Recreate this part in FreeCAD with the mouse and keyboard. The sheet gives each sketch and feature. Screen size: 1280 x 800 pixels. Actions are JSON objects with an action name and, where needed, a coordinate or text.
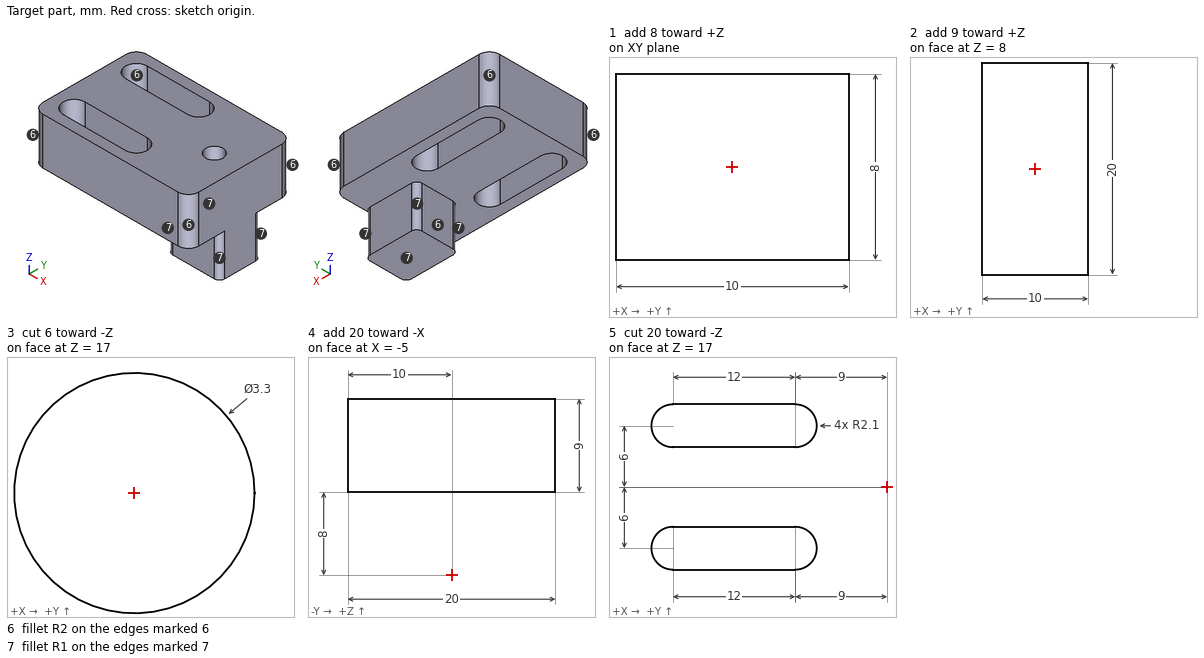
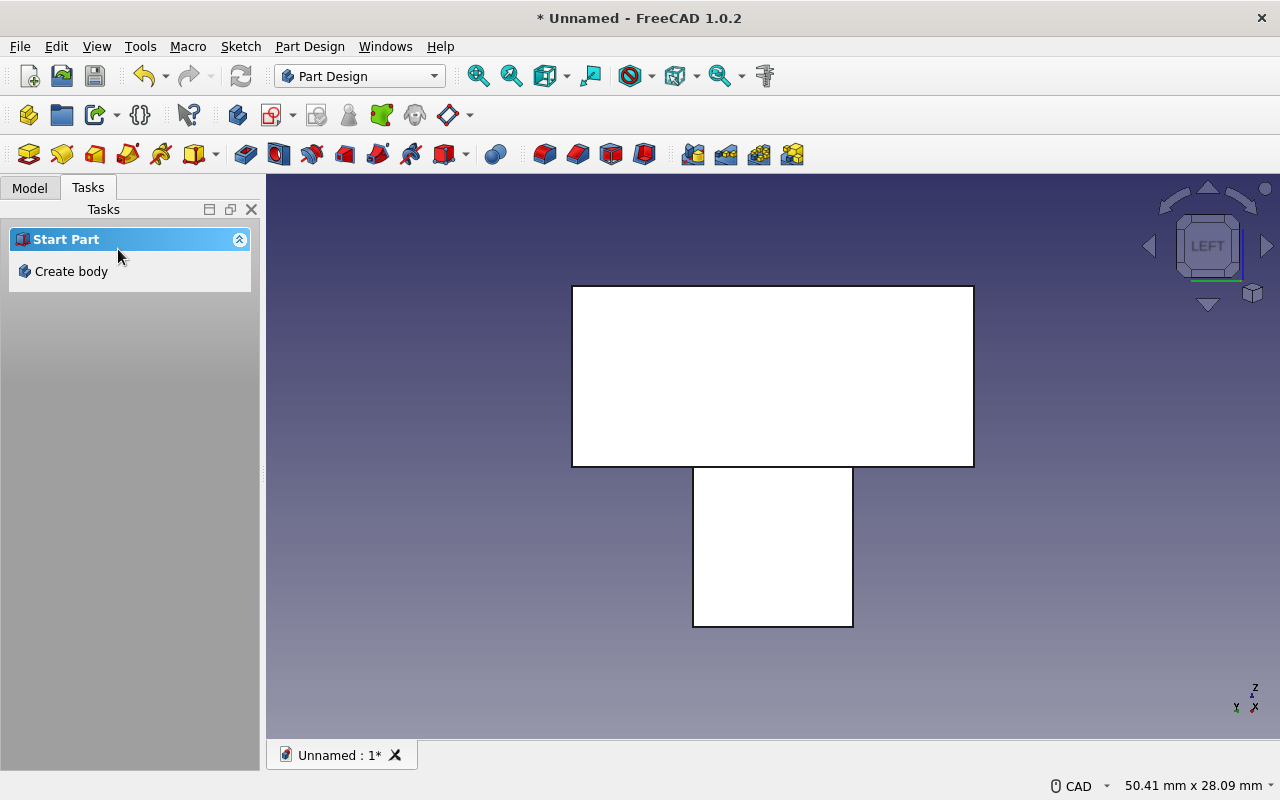
{"action": "key", "text": "0"}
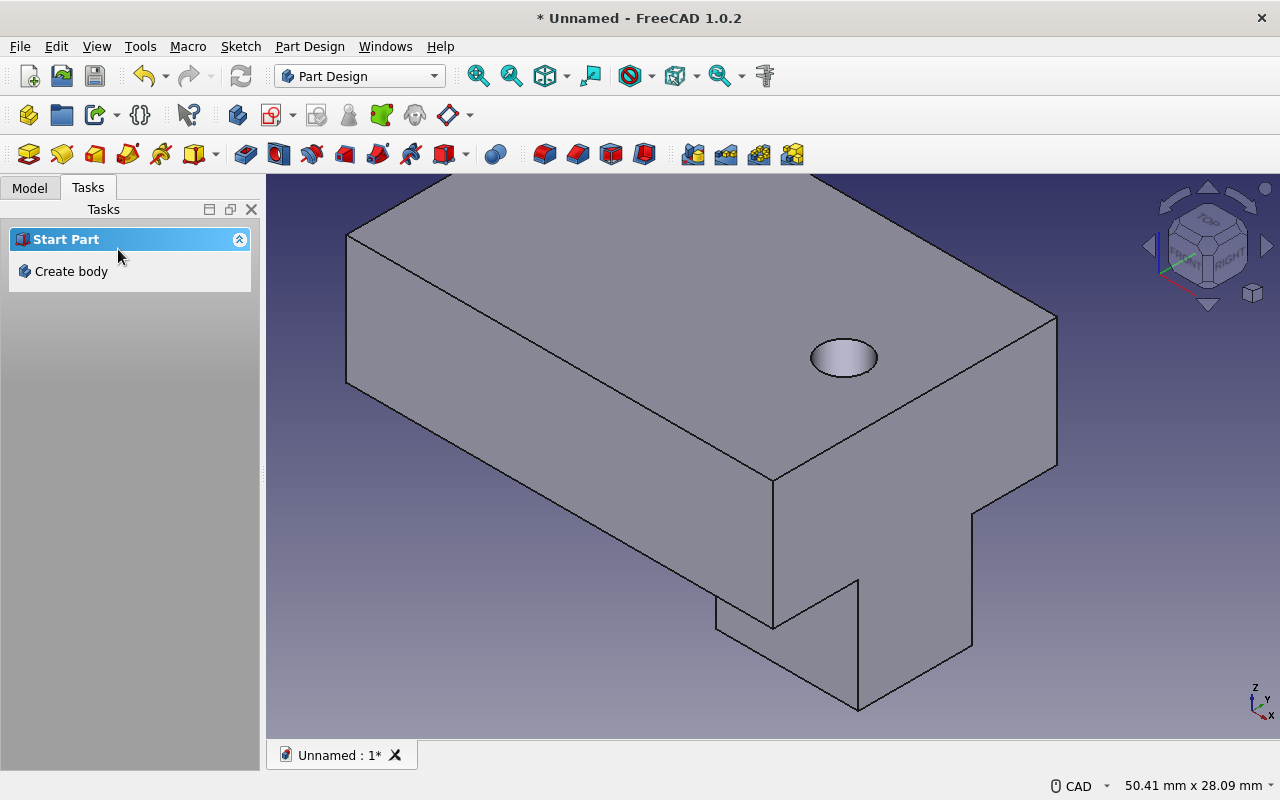
{"action": "left_click", "coordinate": [479, 76]}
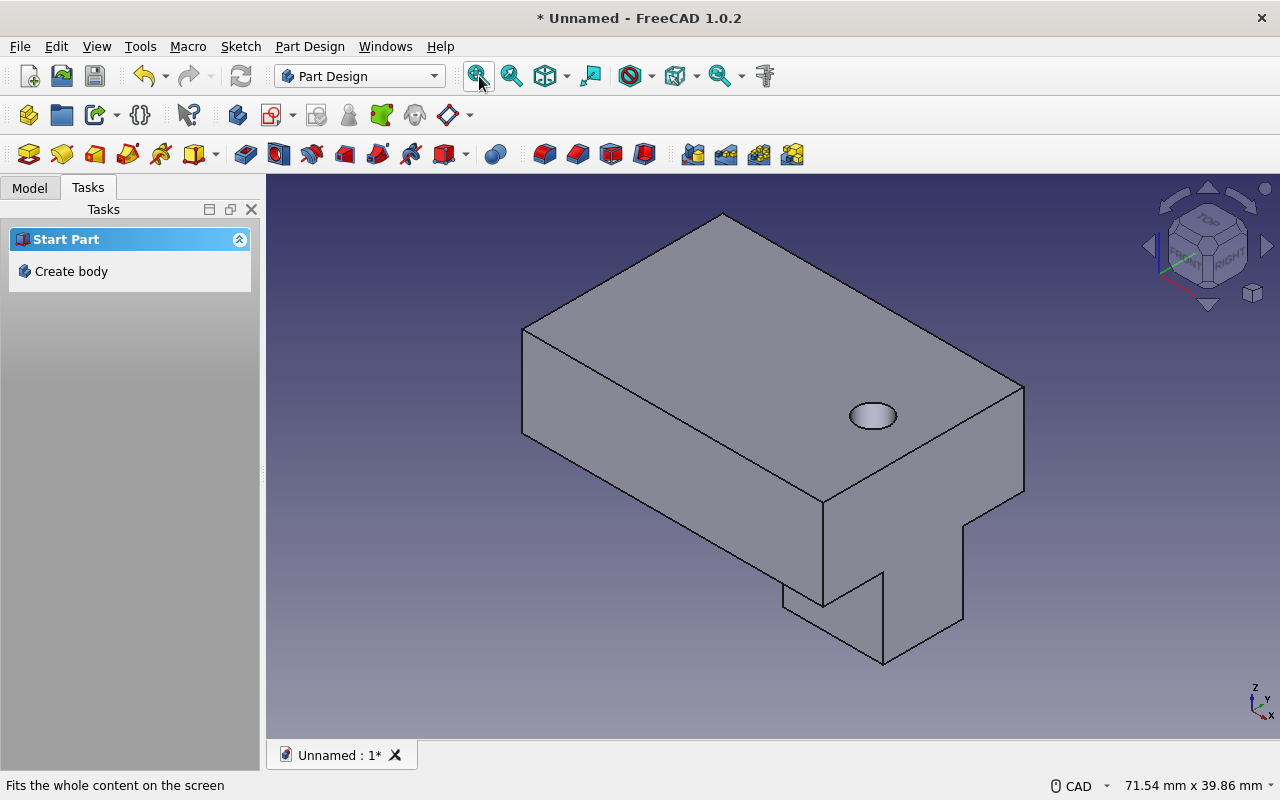
{"action": "left_click", "coordinate": [730, 332]}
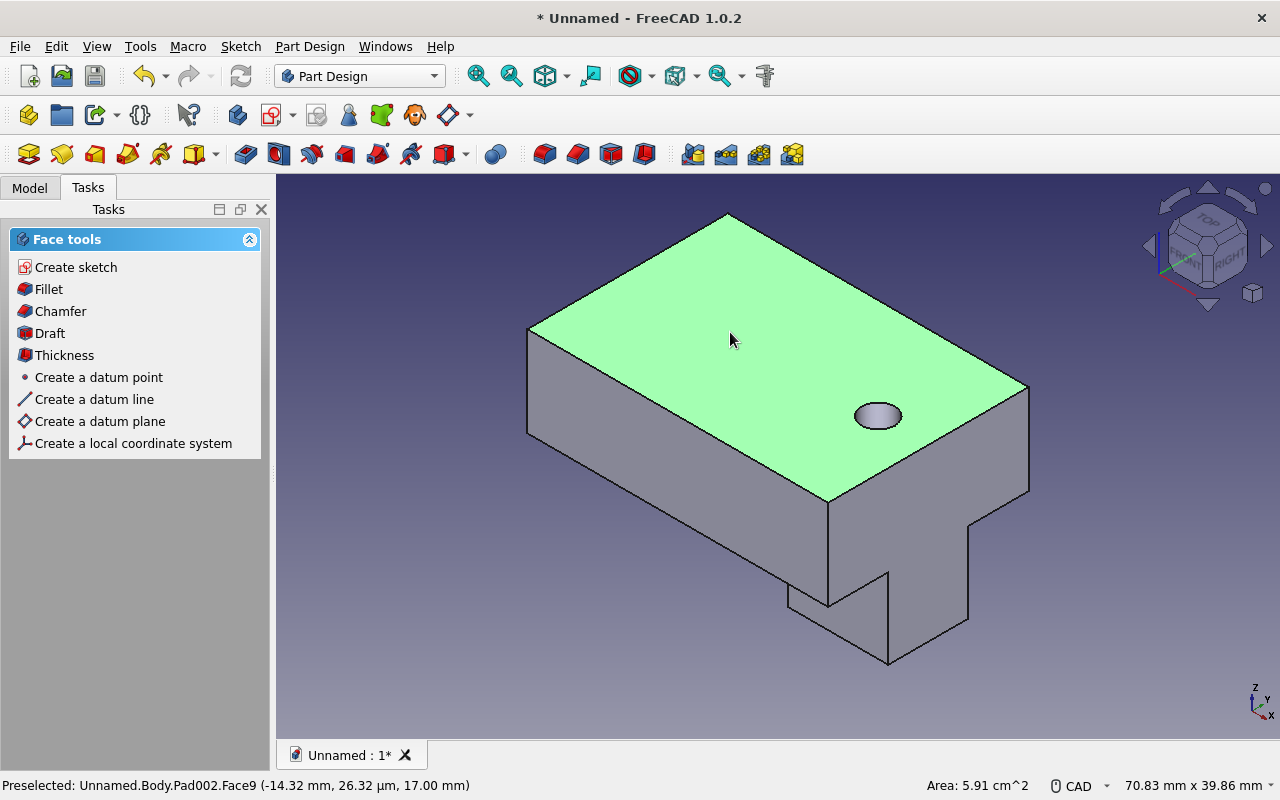
{"action": "left_click", "coordinate": [270, 116]}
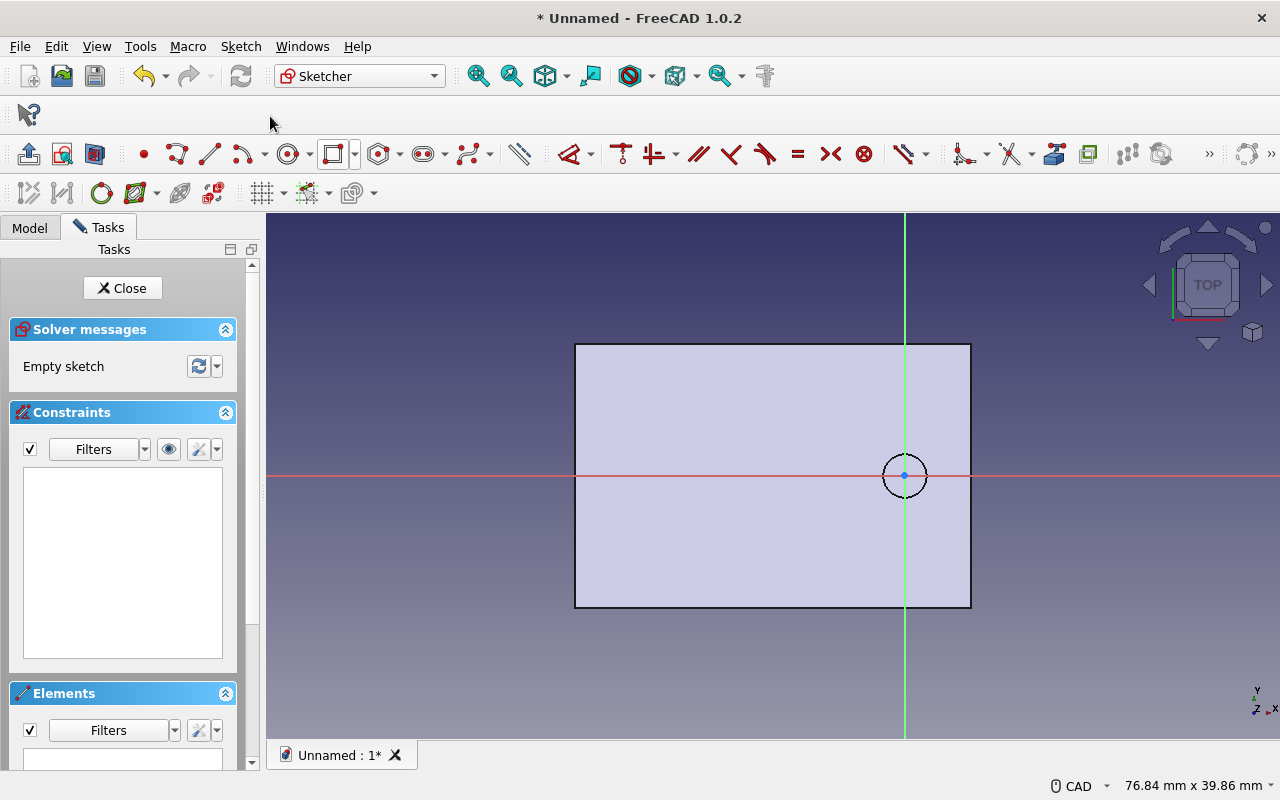
{"action": "scroll", "coordinate": [850, 476], "scroll_direction": "up", "scroll_amount": 2}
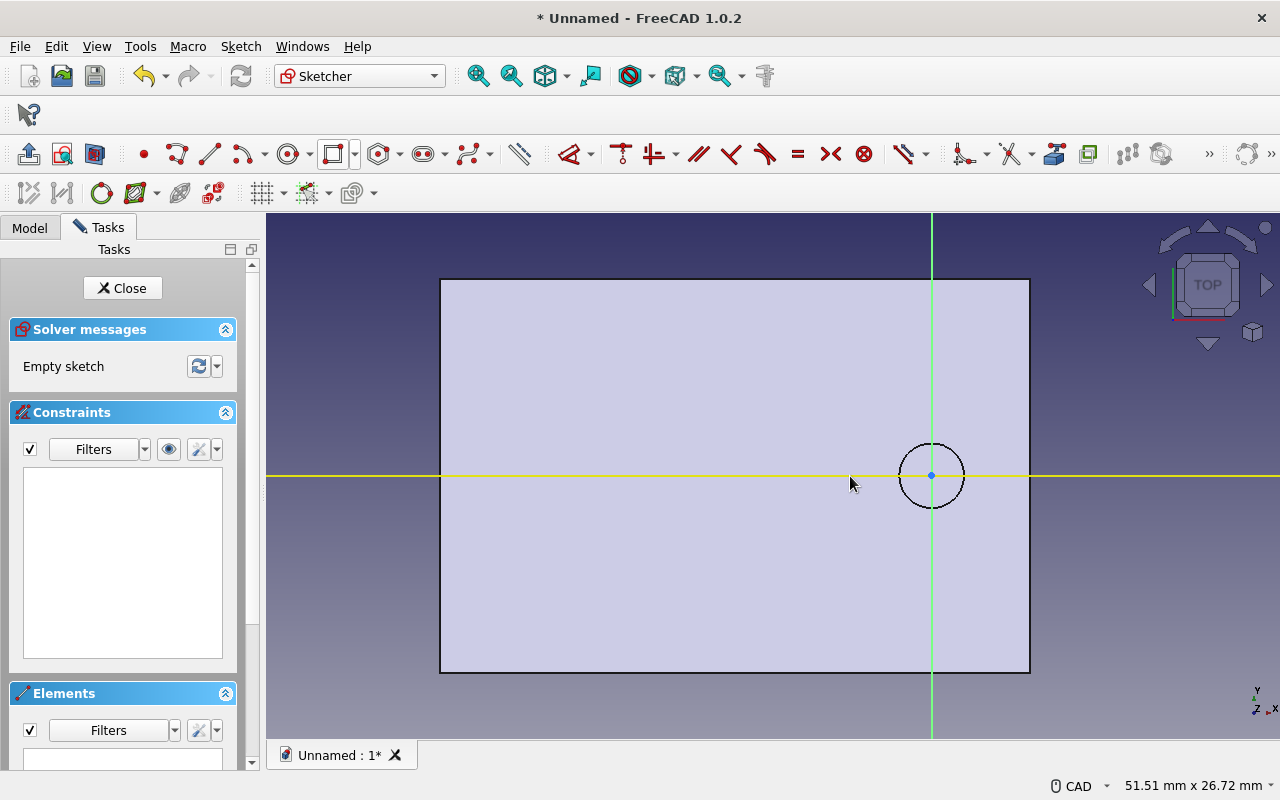
{"action": "left_click", "coordinate": [422, 154]}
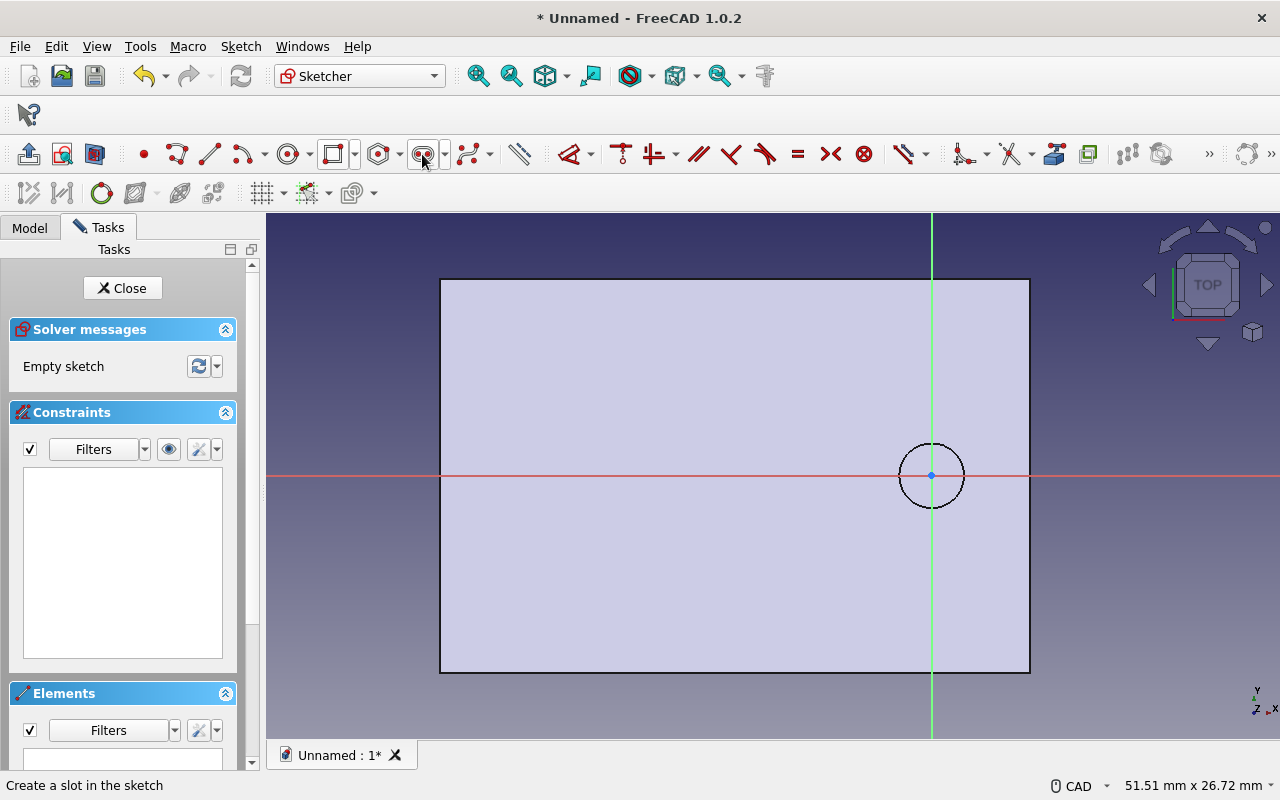
{"action": "left_click", "coordinate": [518, 358]}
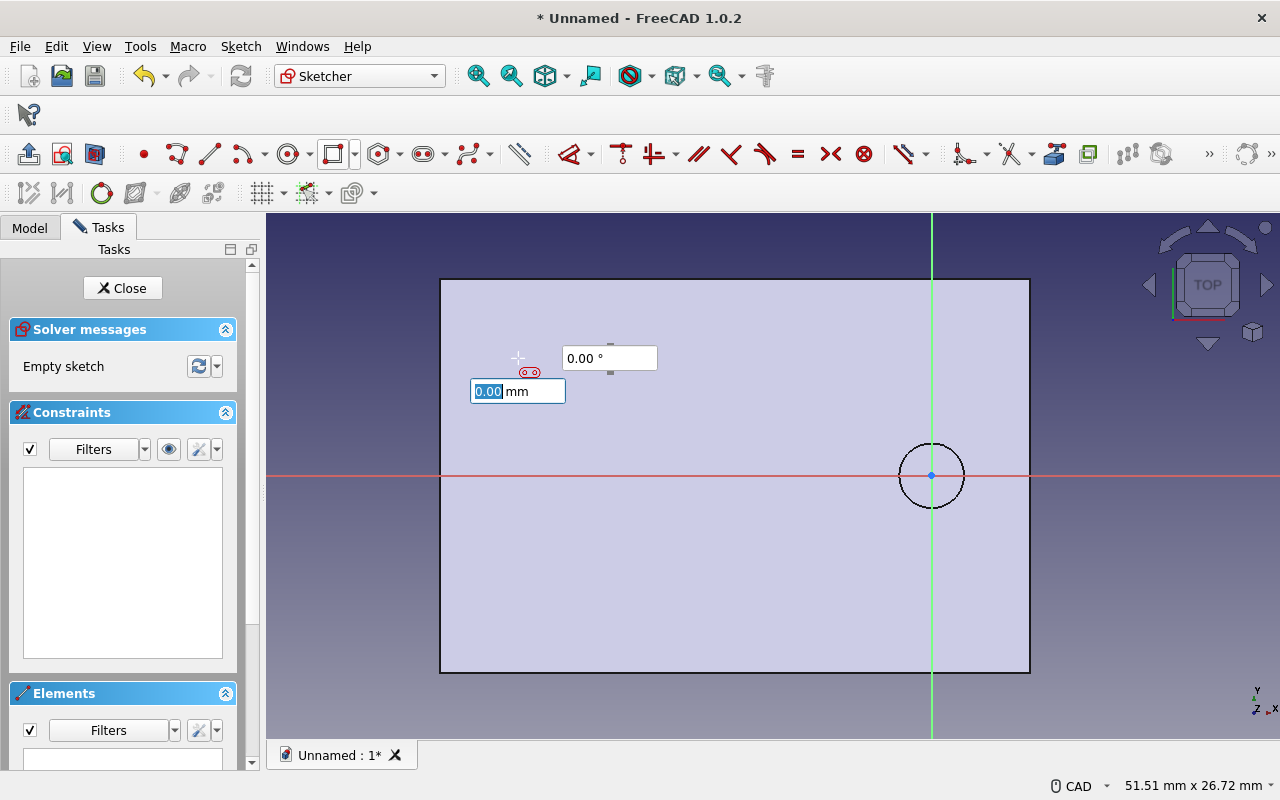
{"action": "left_click", "coordinate": [755, 358]}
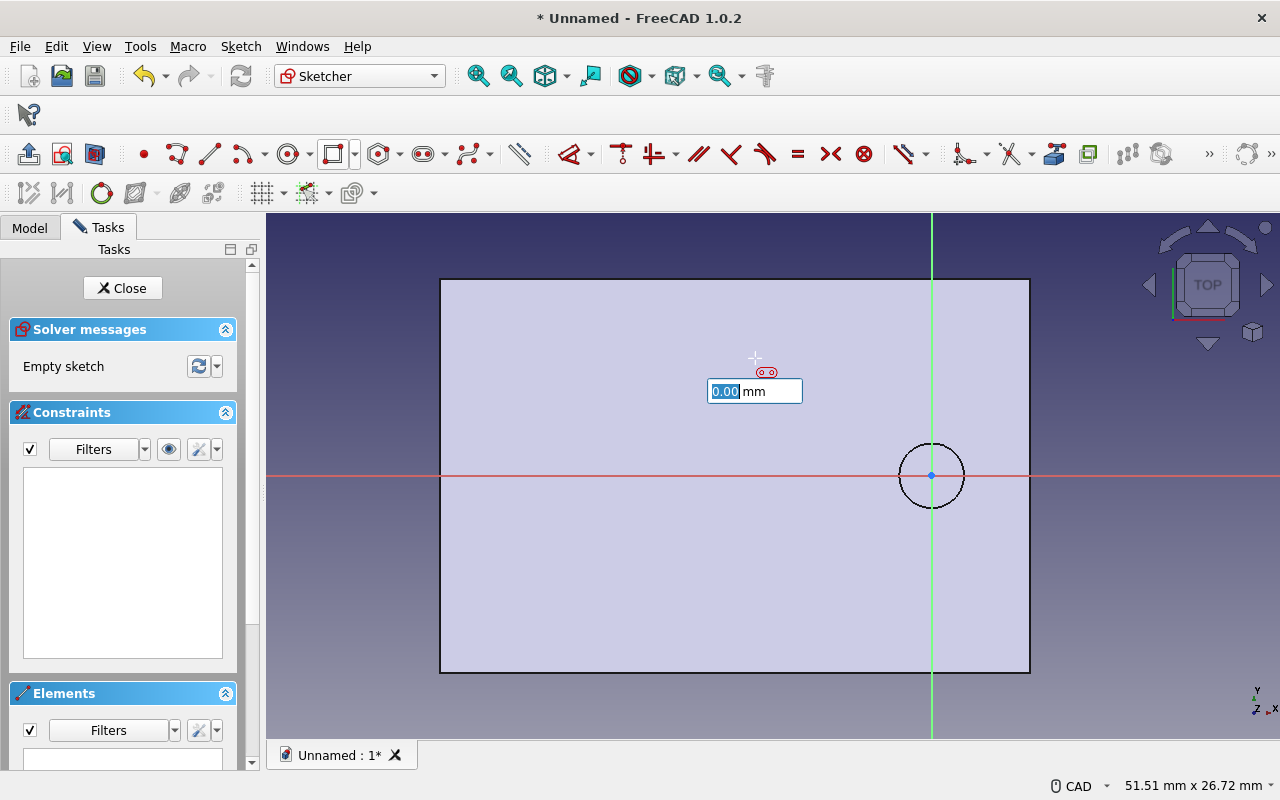
{"action": "left_click", "coordinate": [636, 316]}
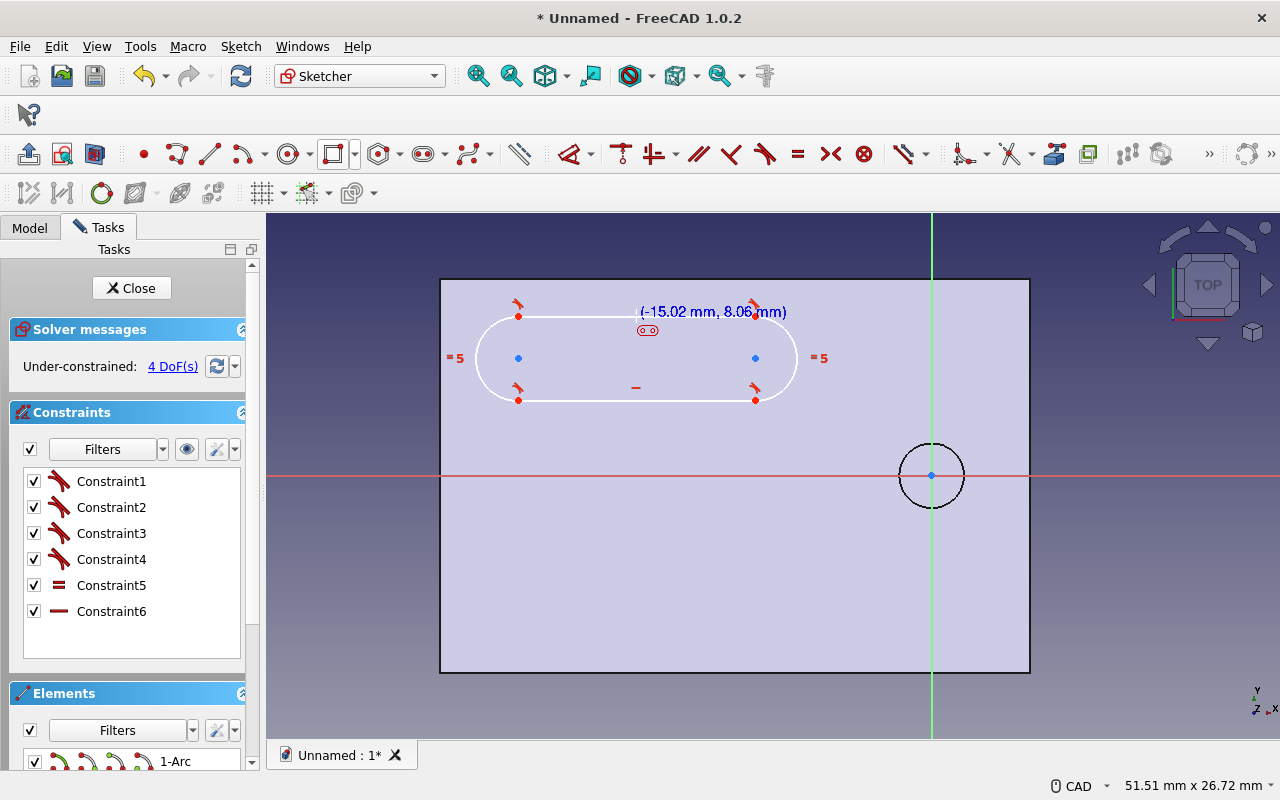
{"action": "left_click", "coordinate": [518, 594]}